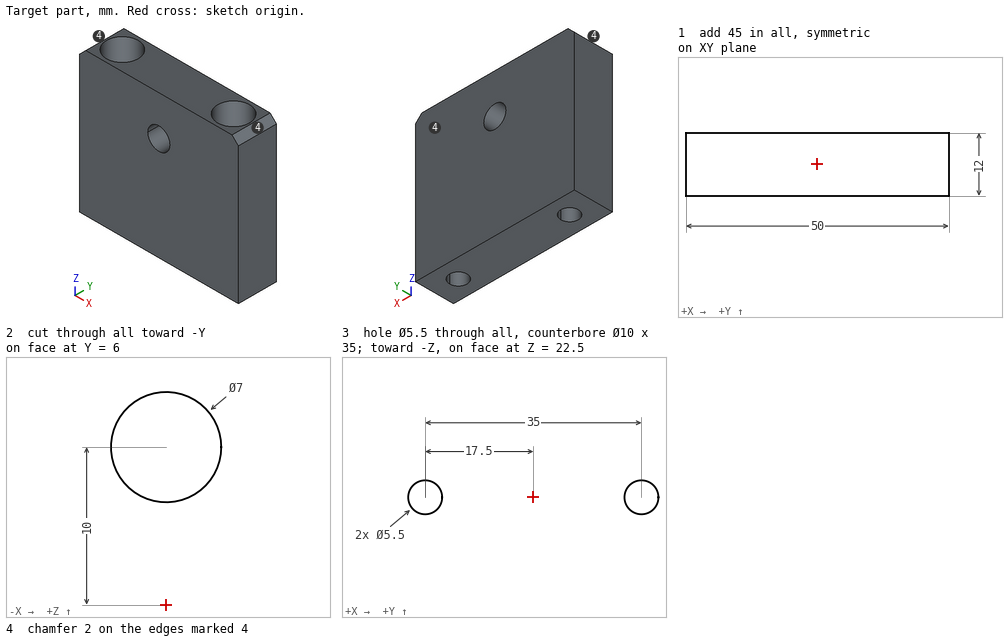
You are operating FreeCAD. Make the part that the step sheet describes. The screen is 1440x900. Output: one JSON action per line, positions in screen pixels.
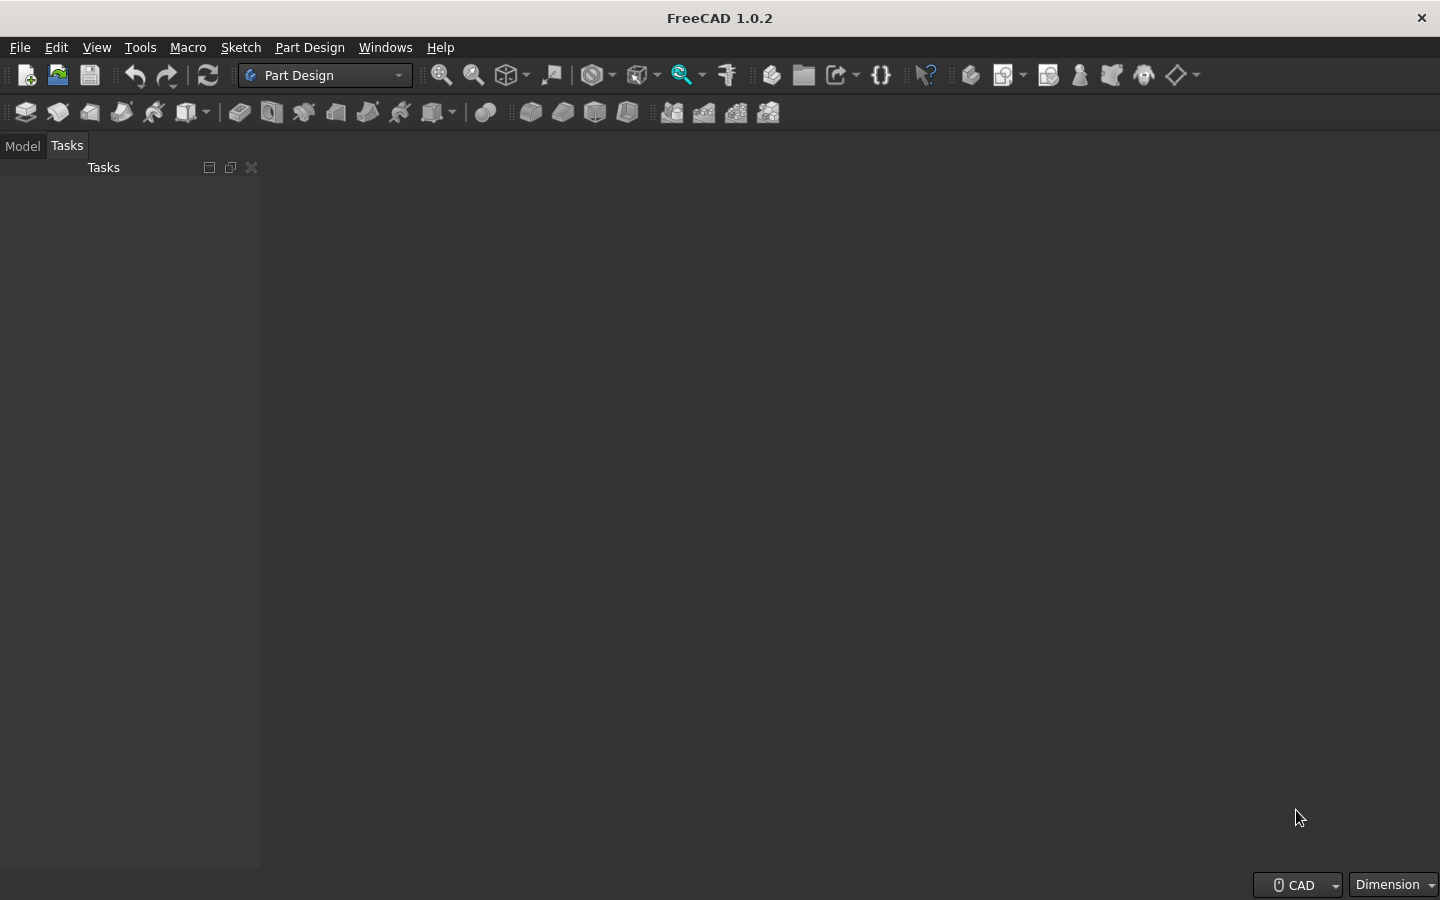
{"action": "key", "text": "ctrl+n"}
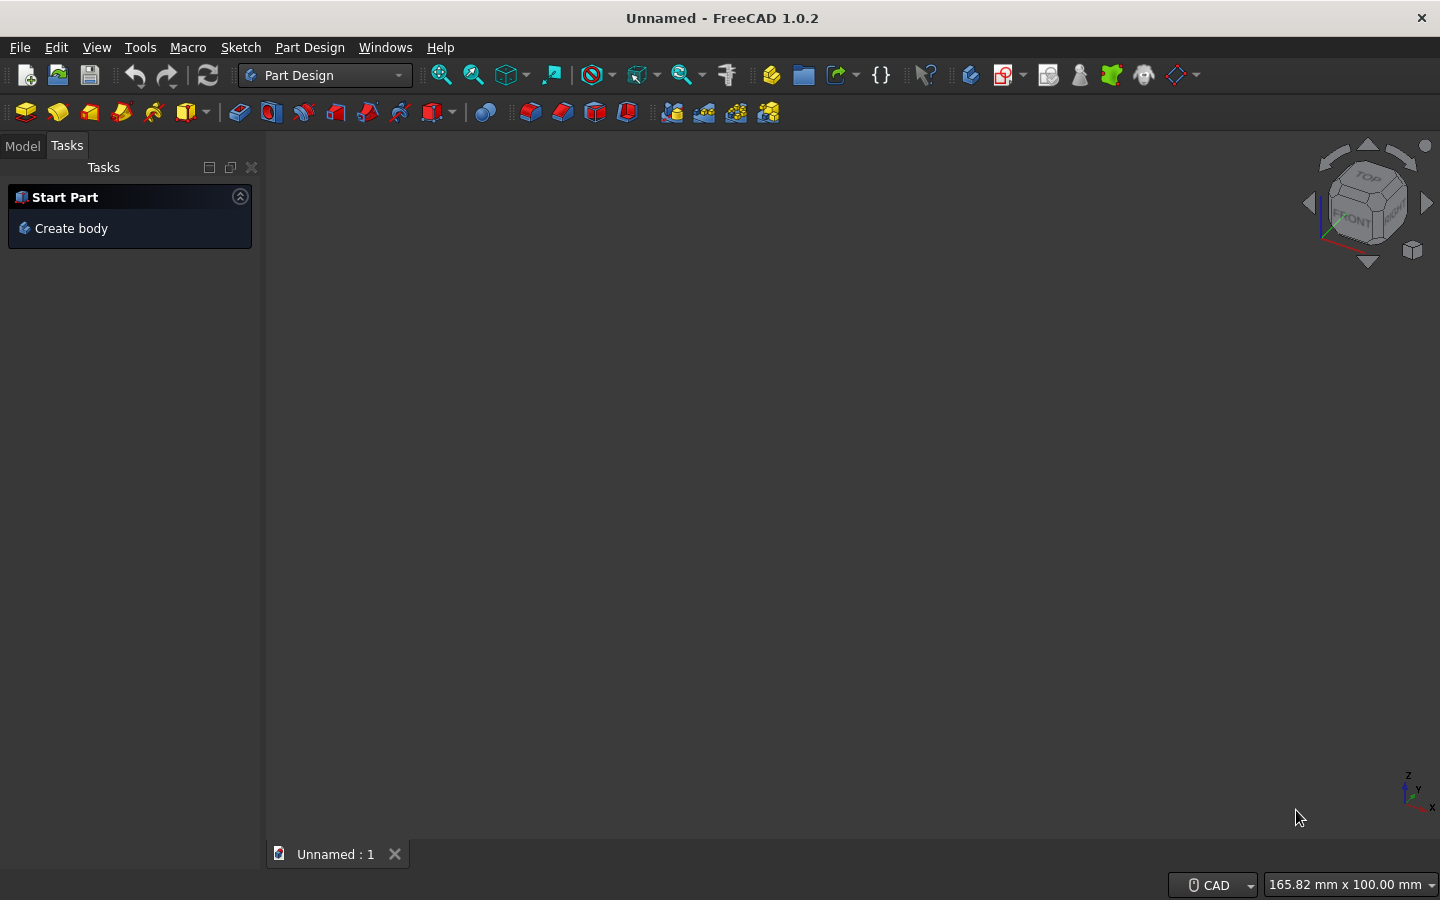
{"action": "left_click", "coordinate": [1004, 76]}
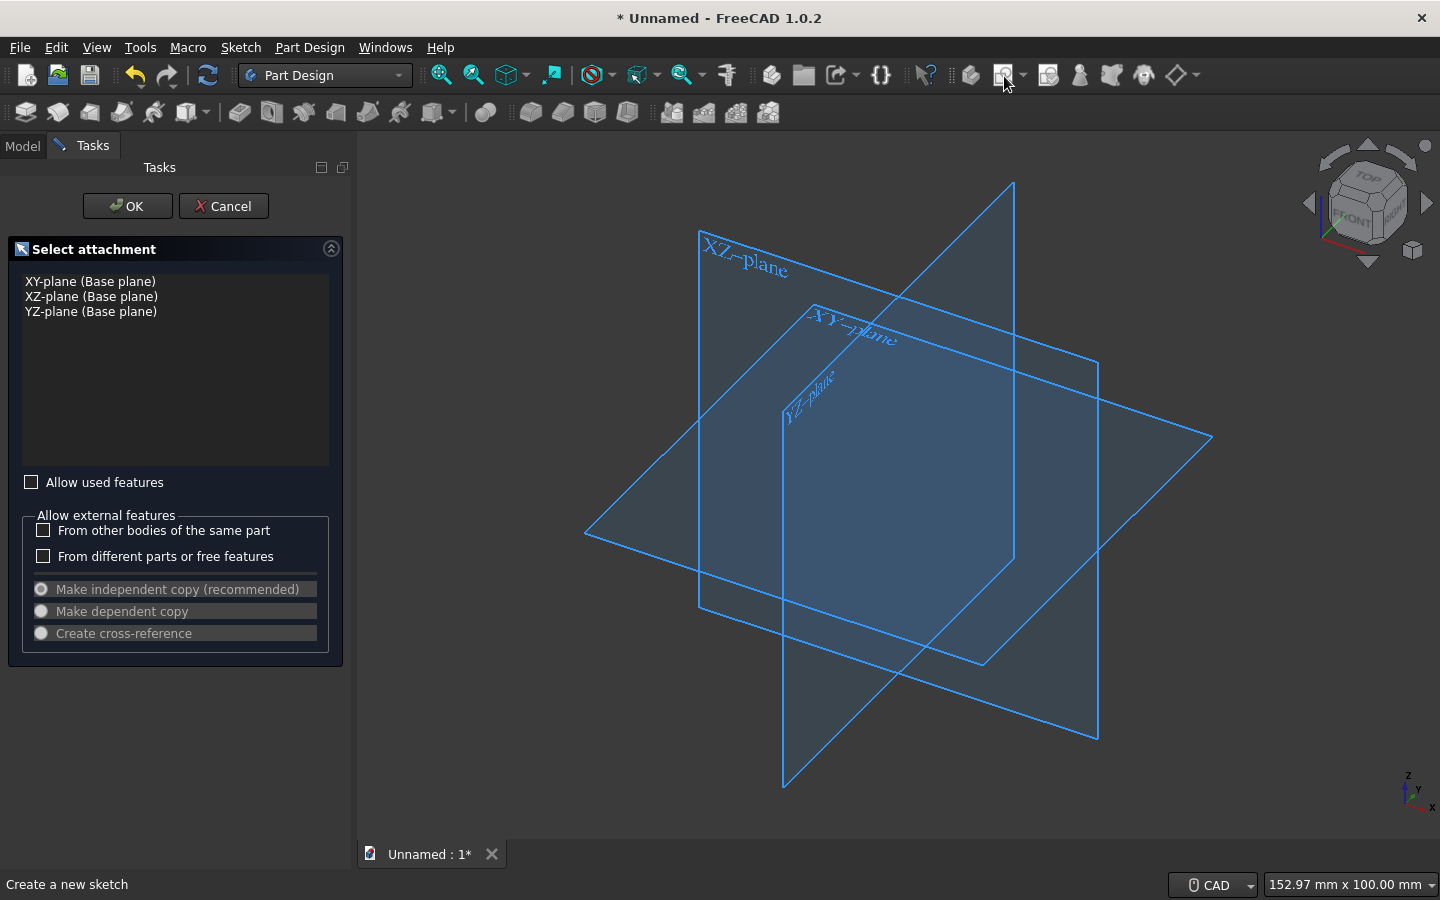
{"action": "left_click", "coordinate": [82, 282]}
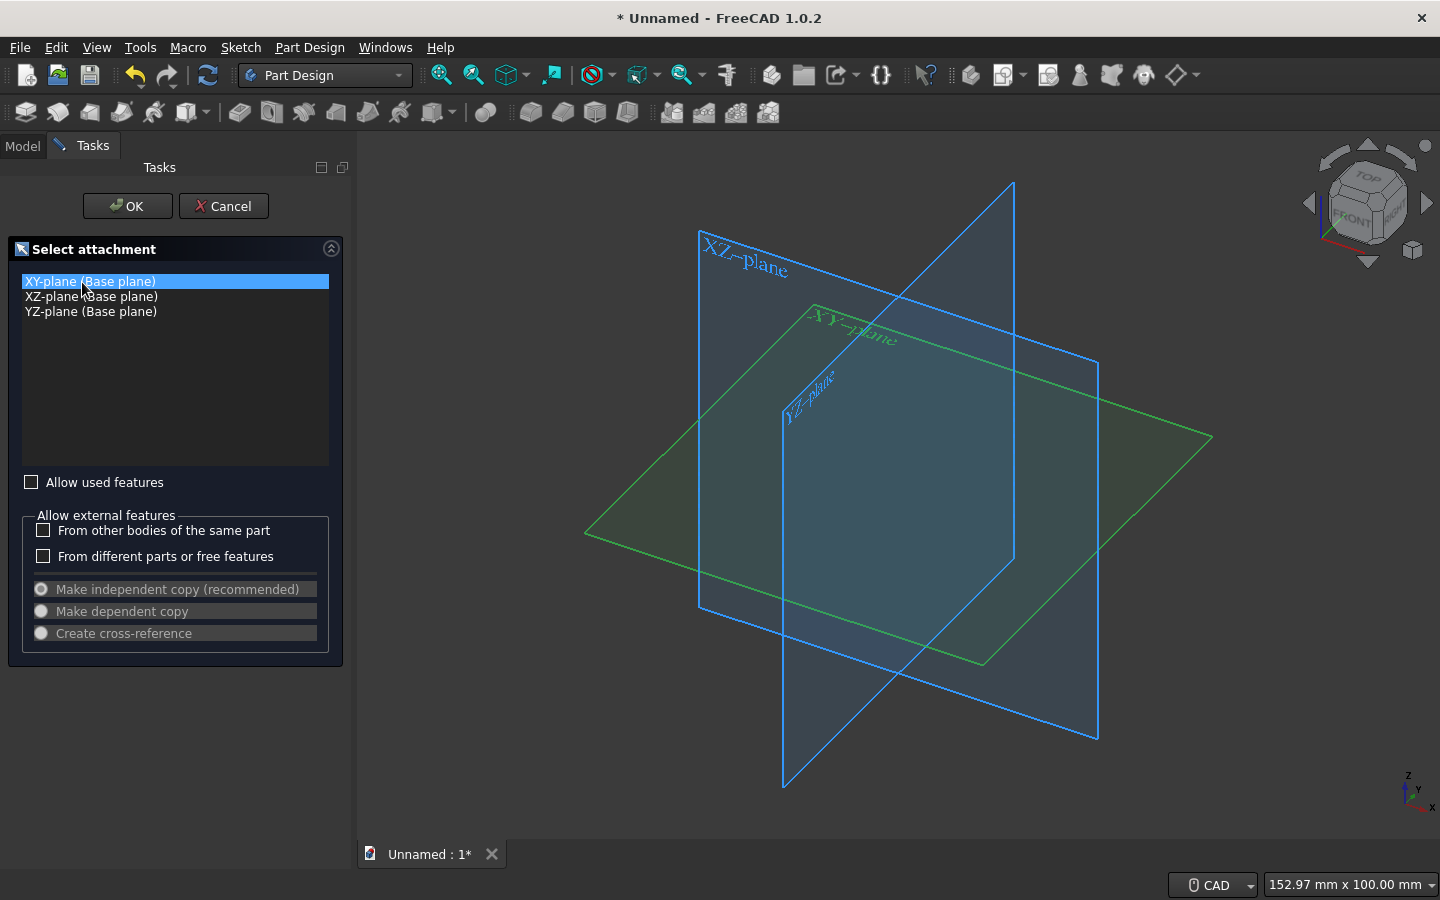
{"action": "left_click", "coordinate": [128, 206]}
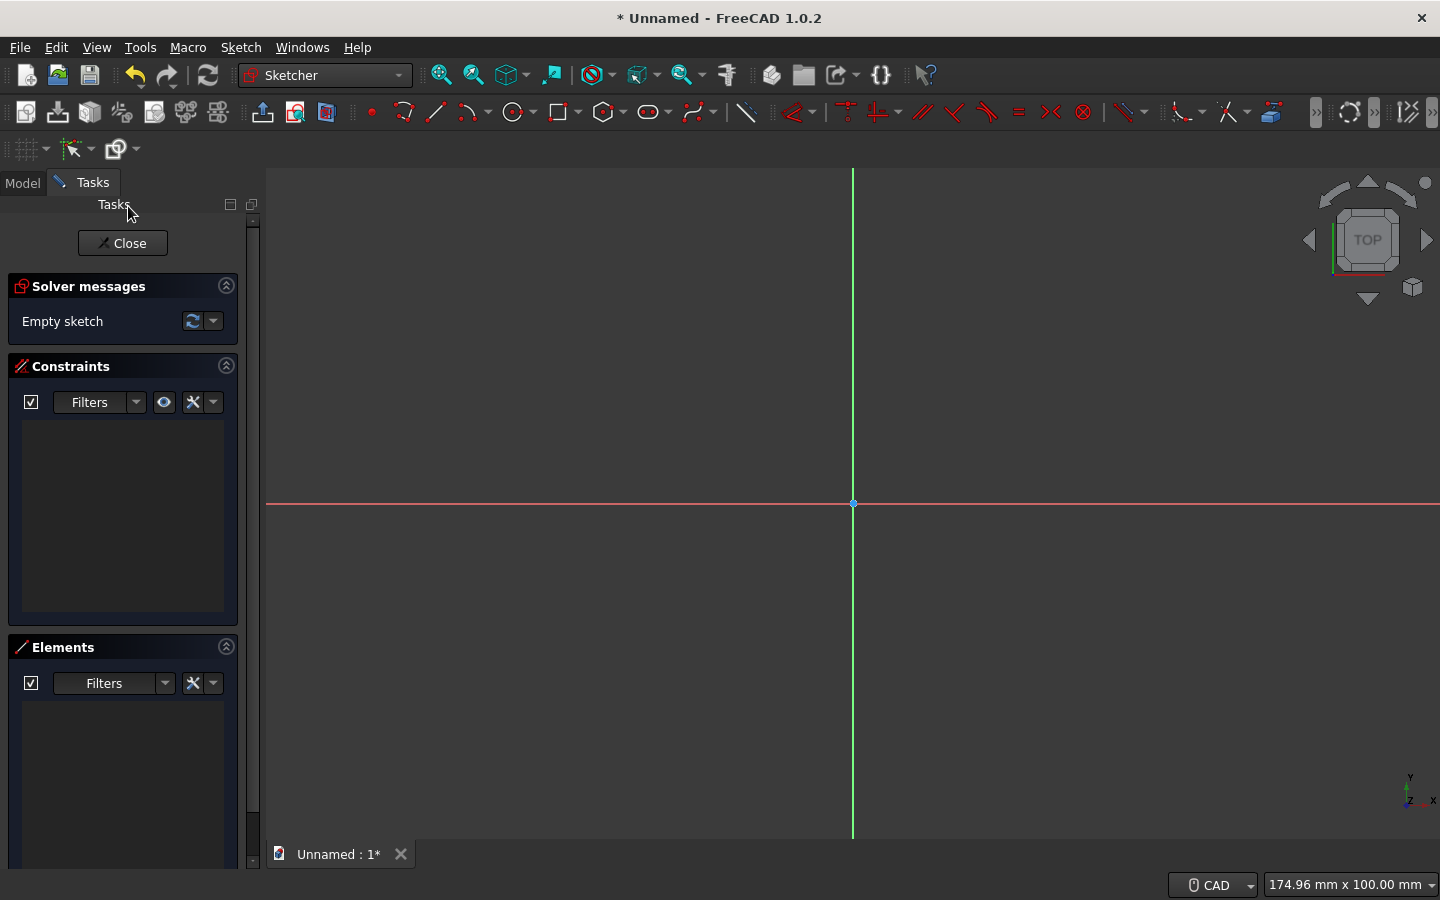
{"action": "scroll", "coordinate": [909, 504], "scroll_direction": "up", "scroll_amount": 4}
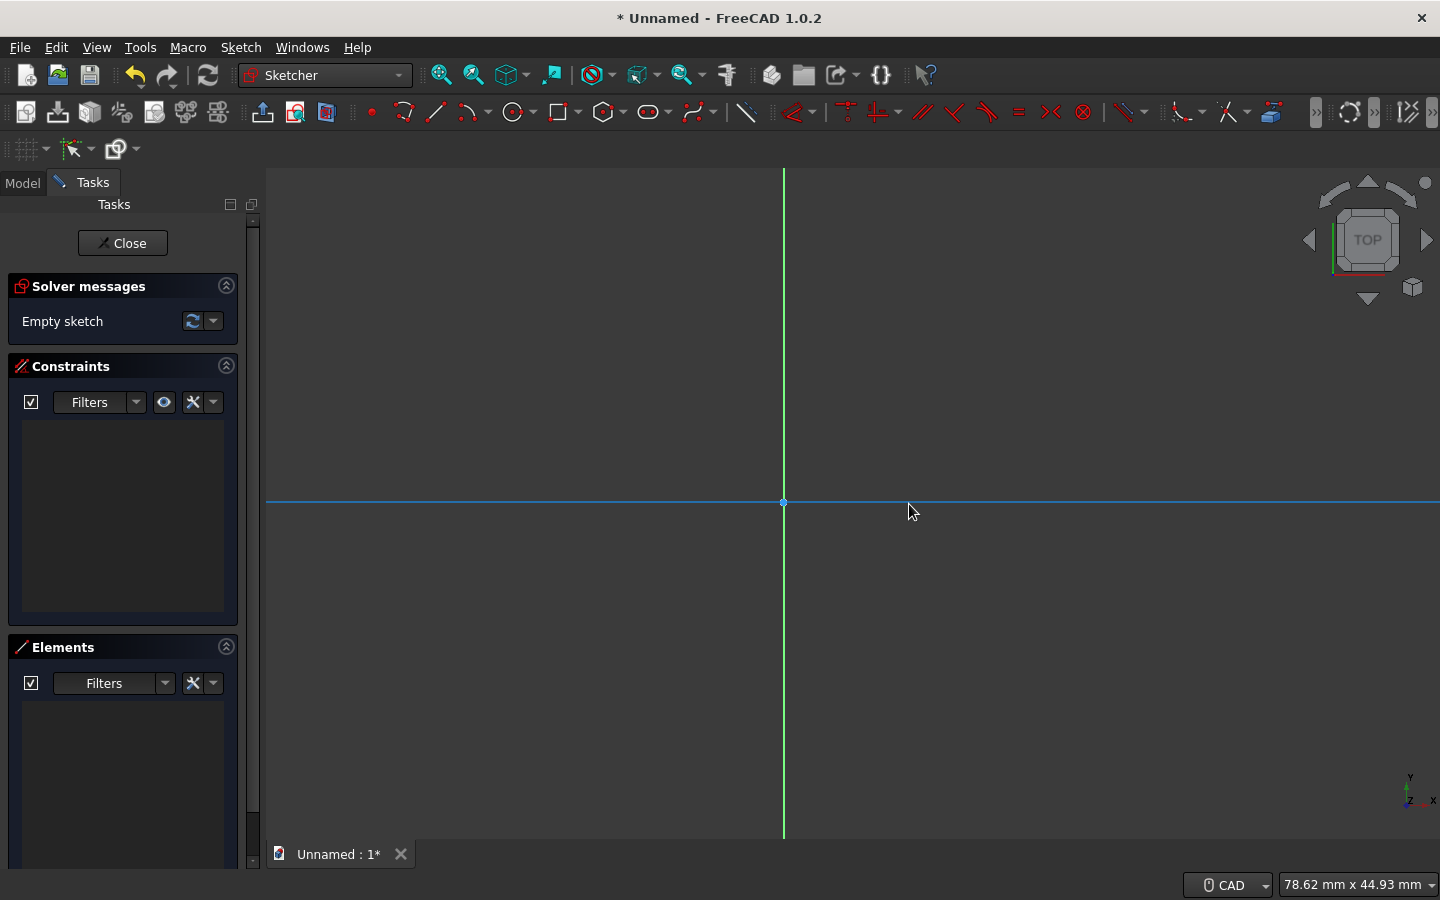
{"action": "key", "text": "g v"}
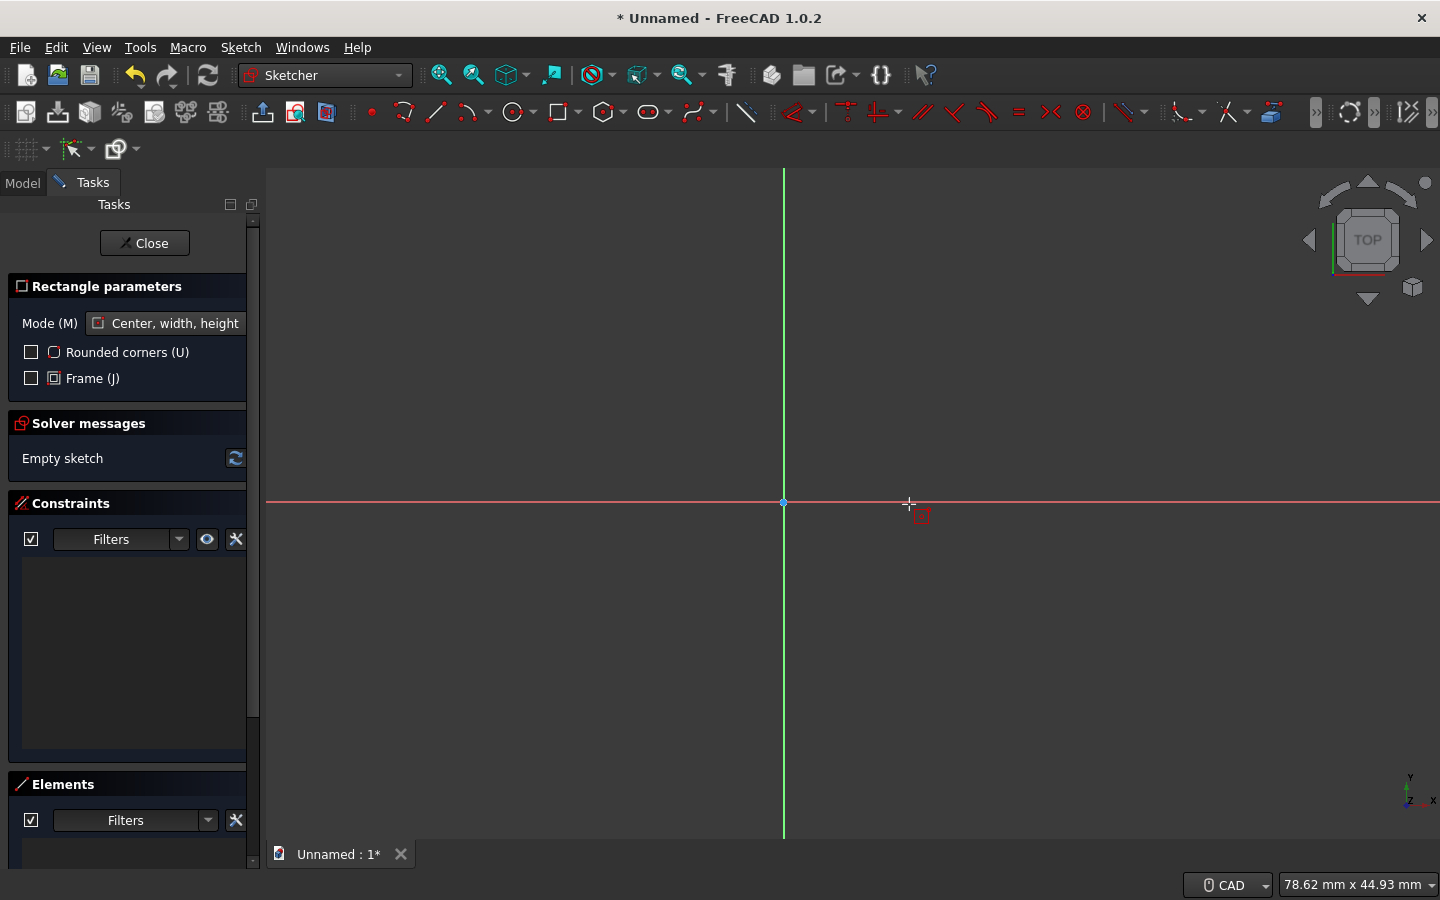
{"action": "left_click", "coordinate": [784, 502]}
{"action": "left_click", "coordinate": [1157, 413]}
{"action": "key", "text": "Escape"}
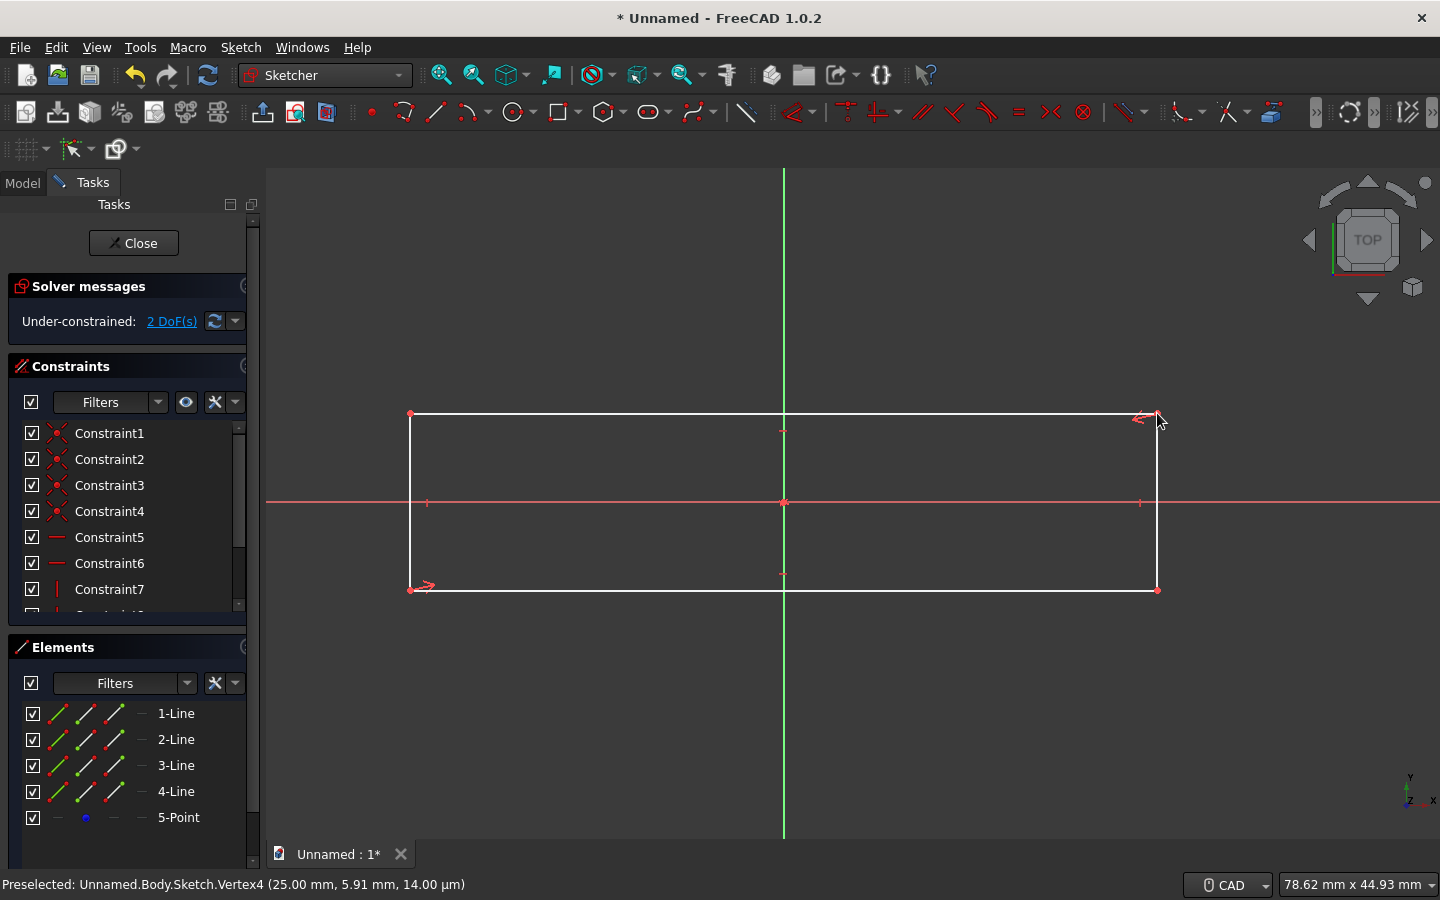
{"action": "key", "text": "d"}